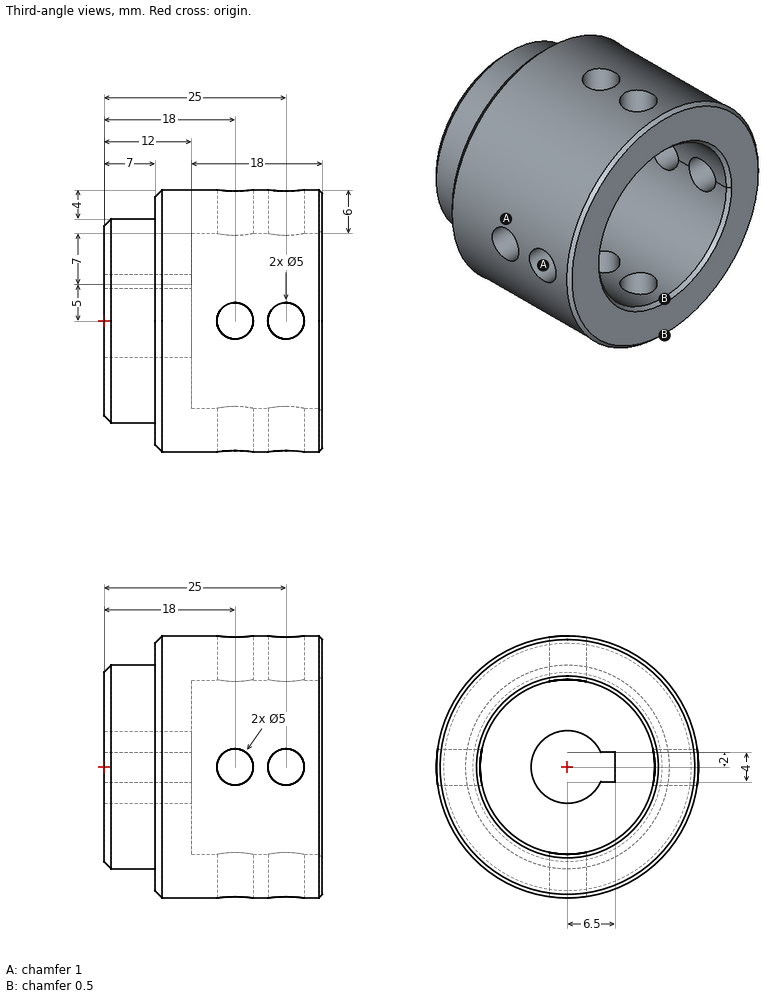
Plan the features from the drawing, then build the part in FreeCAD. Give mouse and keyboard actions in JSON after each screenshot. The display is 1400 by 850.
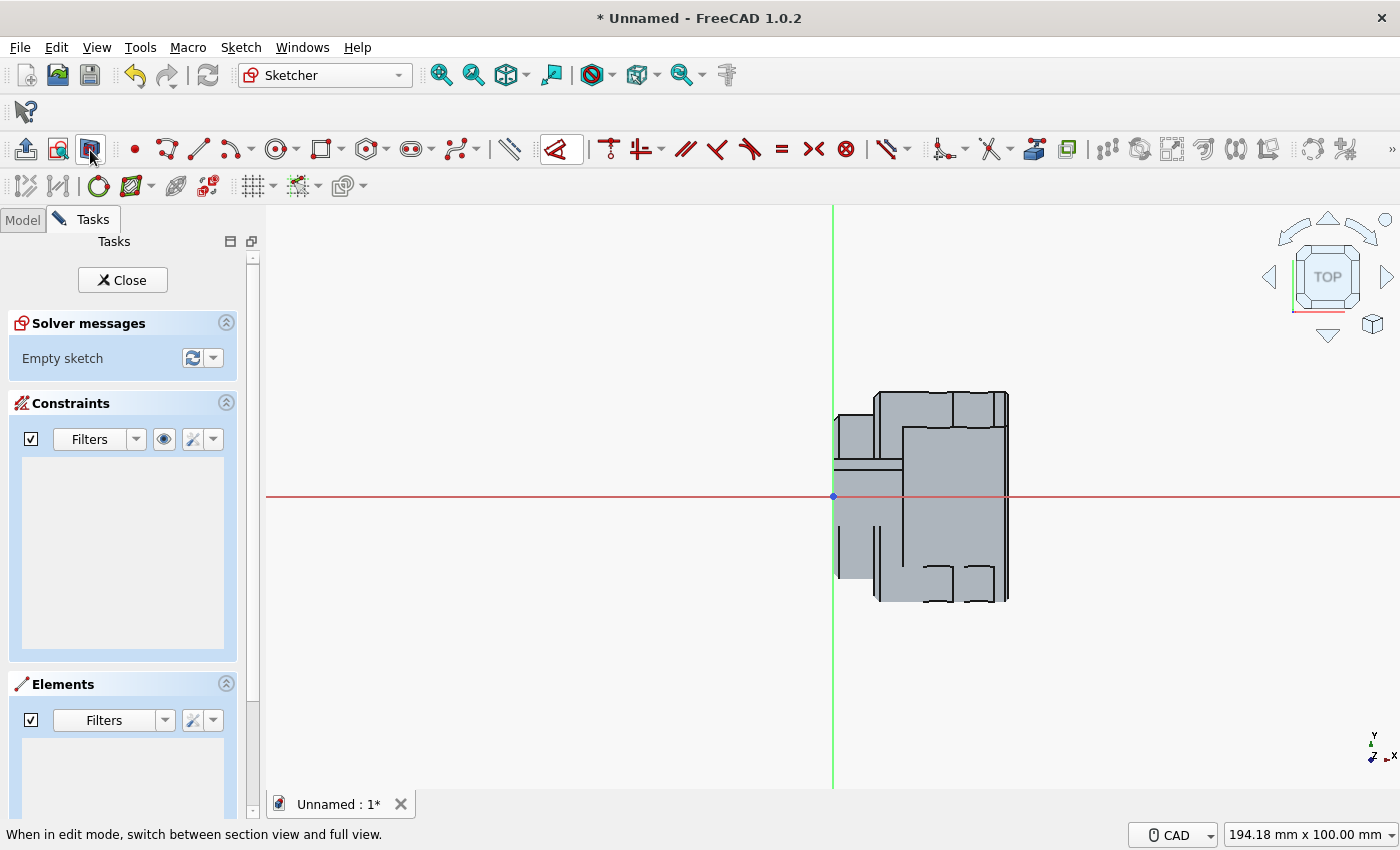
{"action": "scroll", "coordinate": [962, 497], "scroll_direction": "up", "scroll_amount": 7}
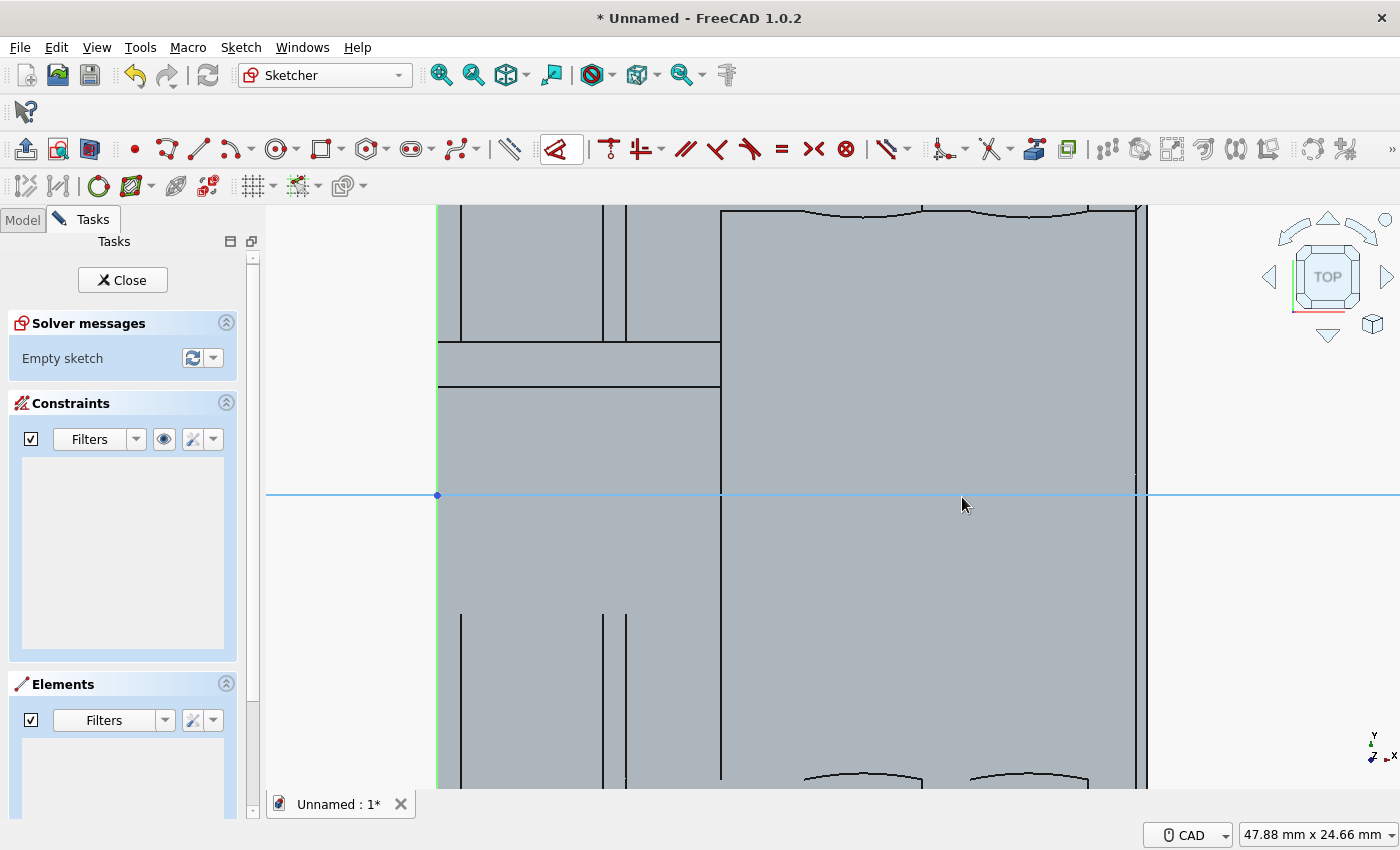
{"action": "left_click", "coordinate": [276, 150]}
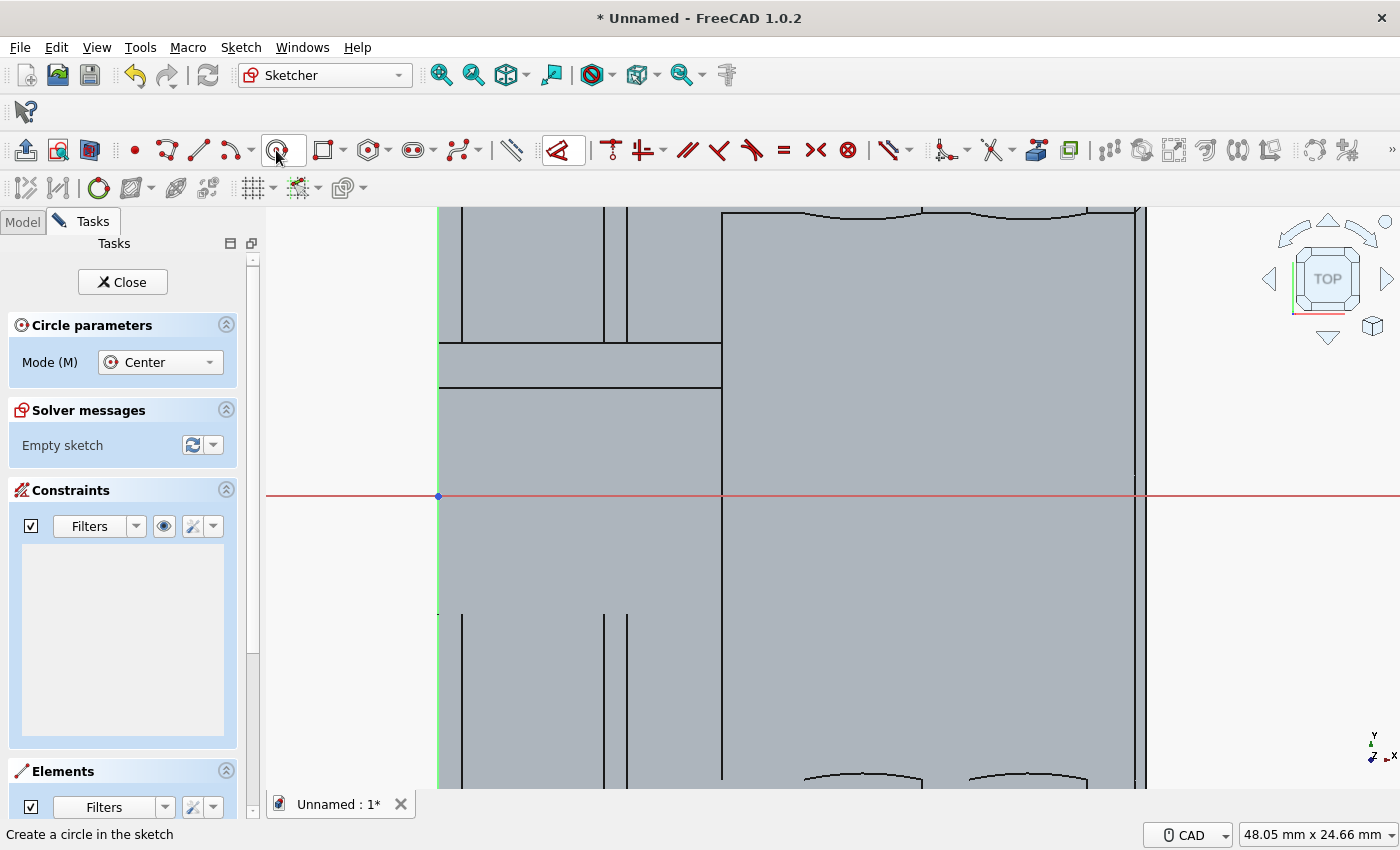
{"action": "left_click", "coordinate": [1028, 496]}
{"action": "left_click", "coordinate": [1070, 455]}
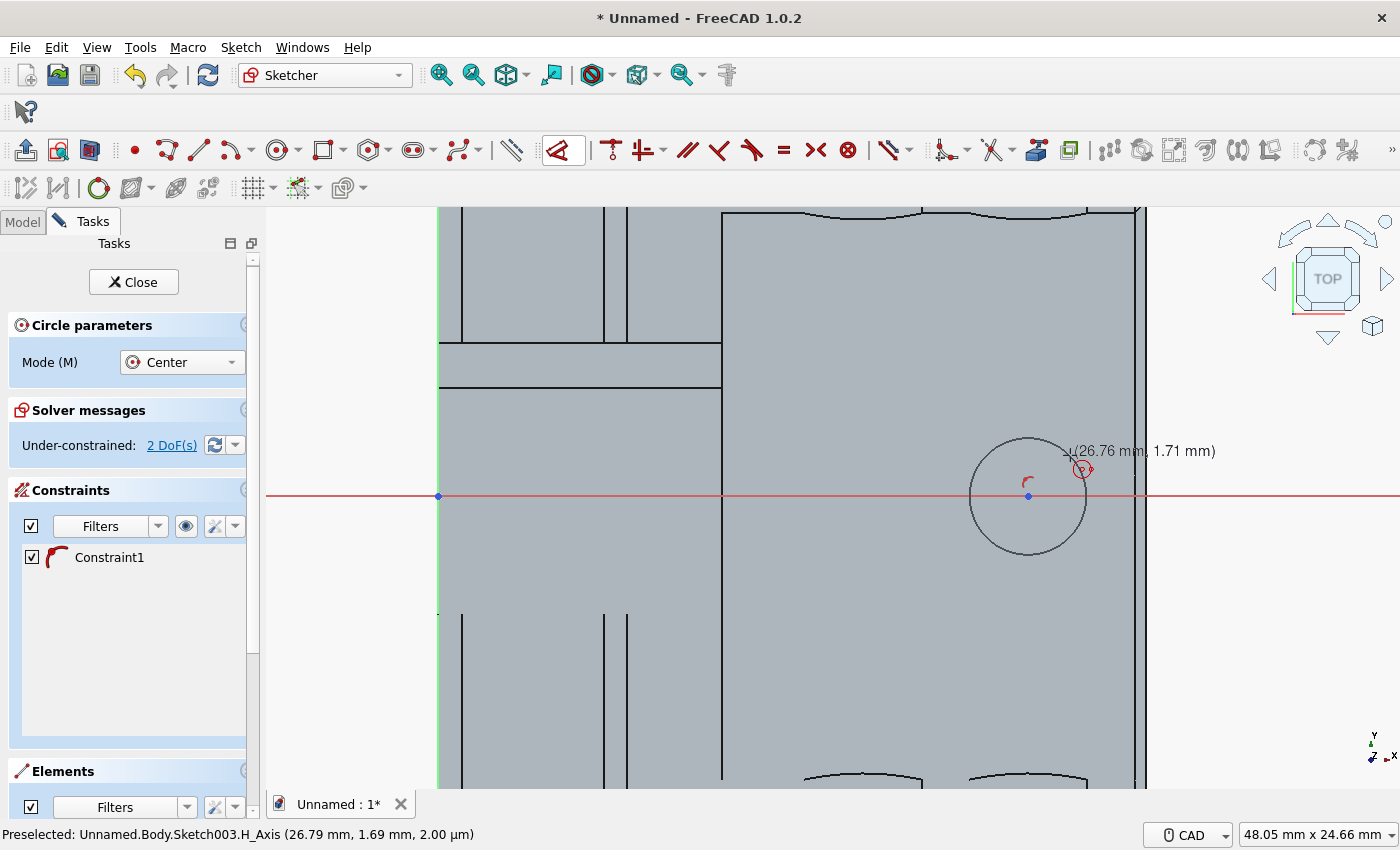
{"action": "left_click", "coordinate": [863, 496]}
{"action": "left_click", "coordinate": [905, 455]}
{"action": "key", "text": "Escape"}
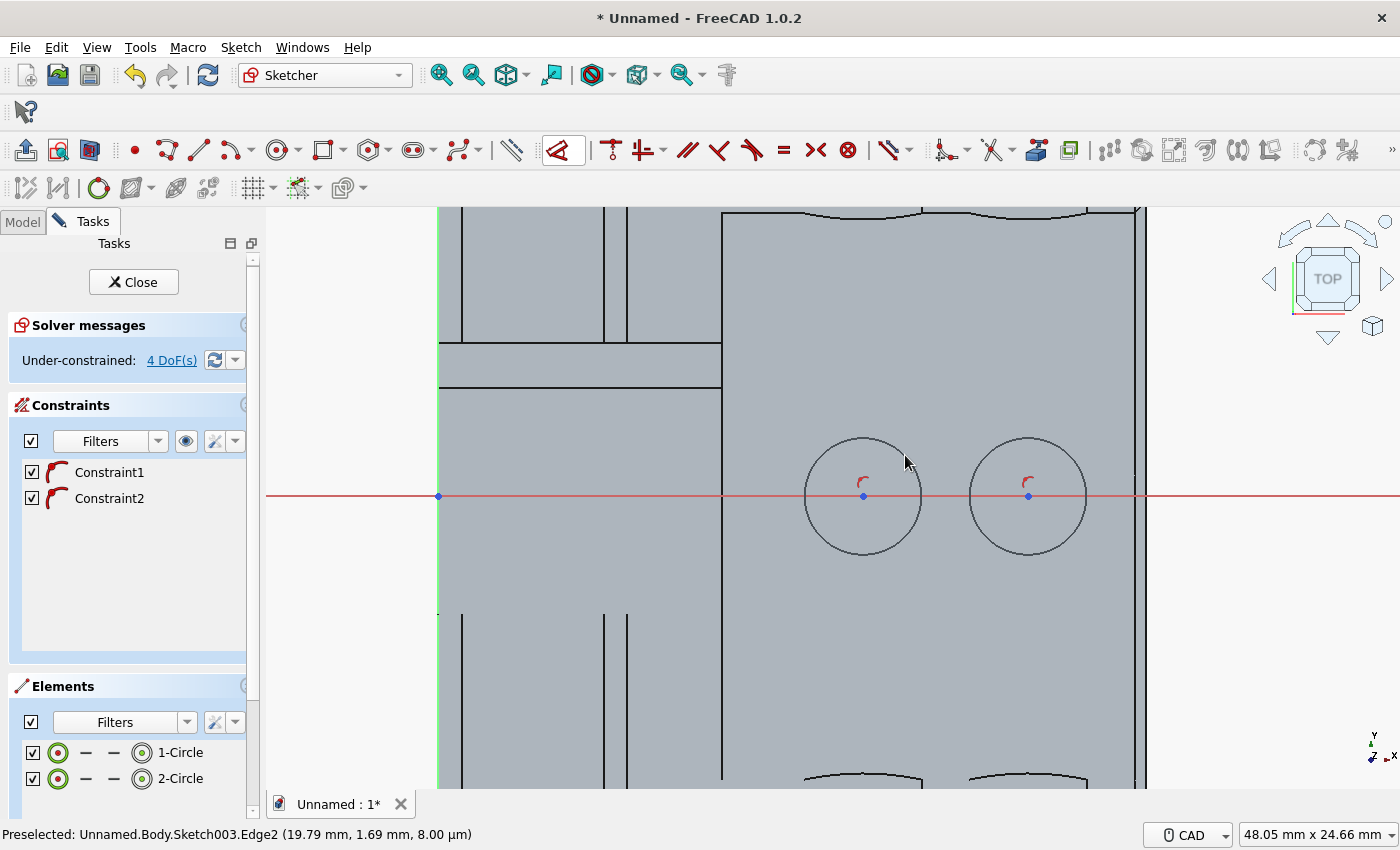
{"action": "left_click", "coordinate": [1069, 455]}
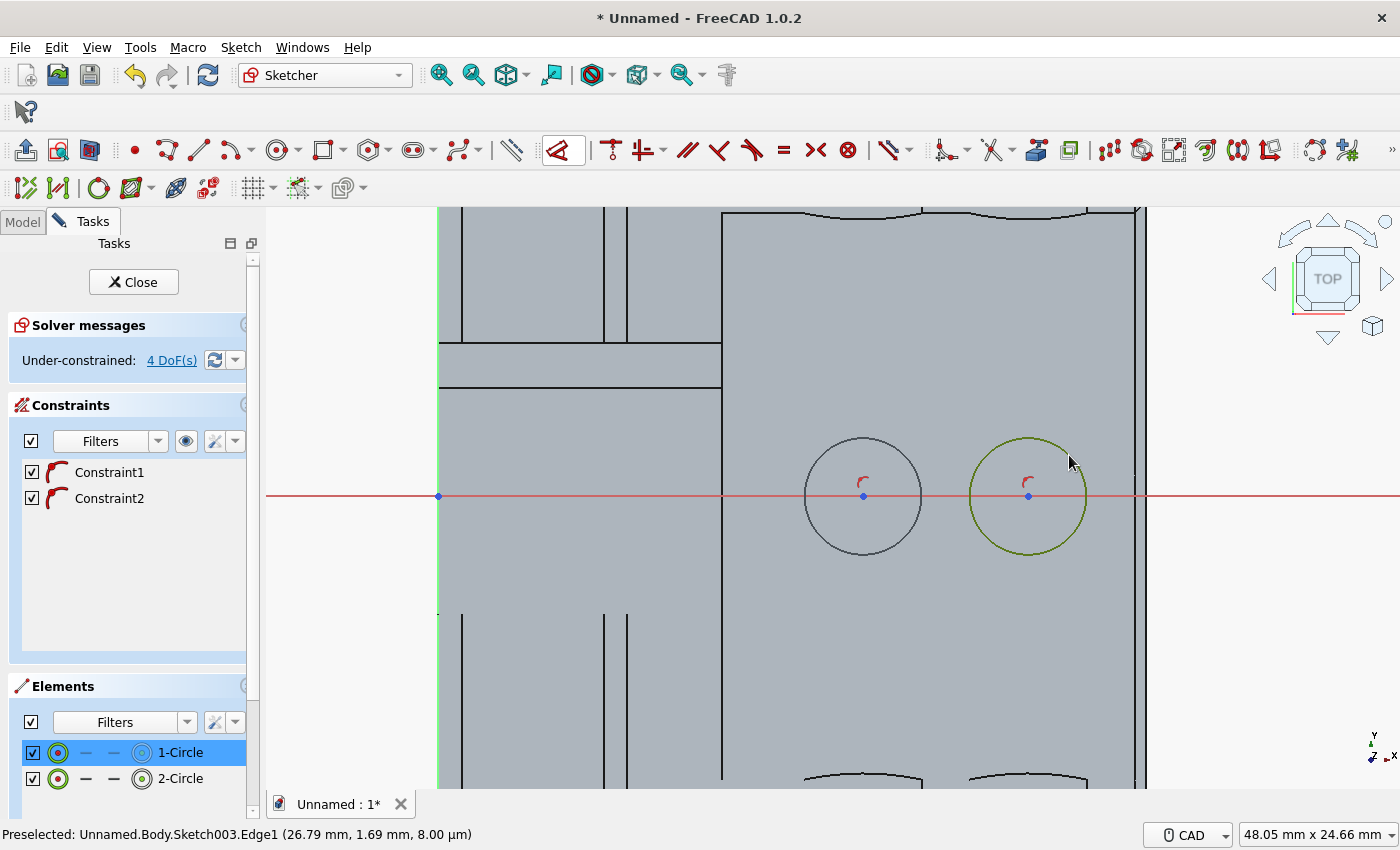
{"action": "left_click", "coordinate": [904, 455]}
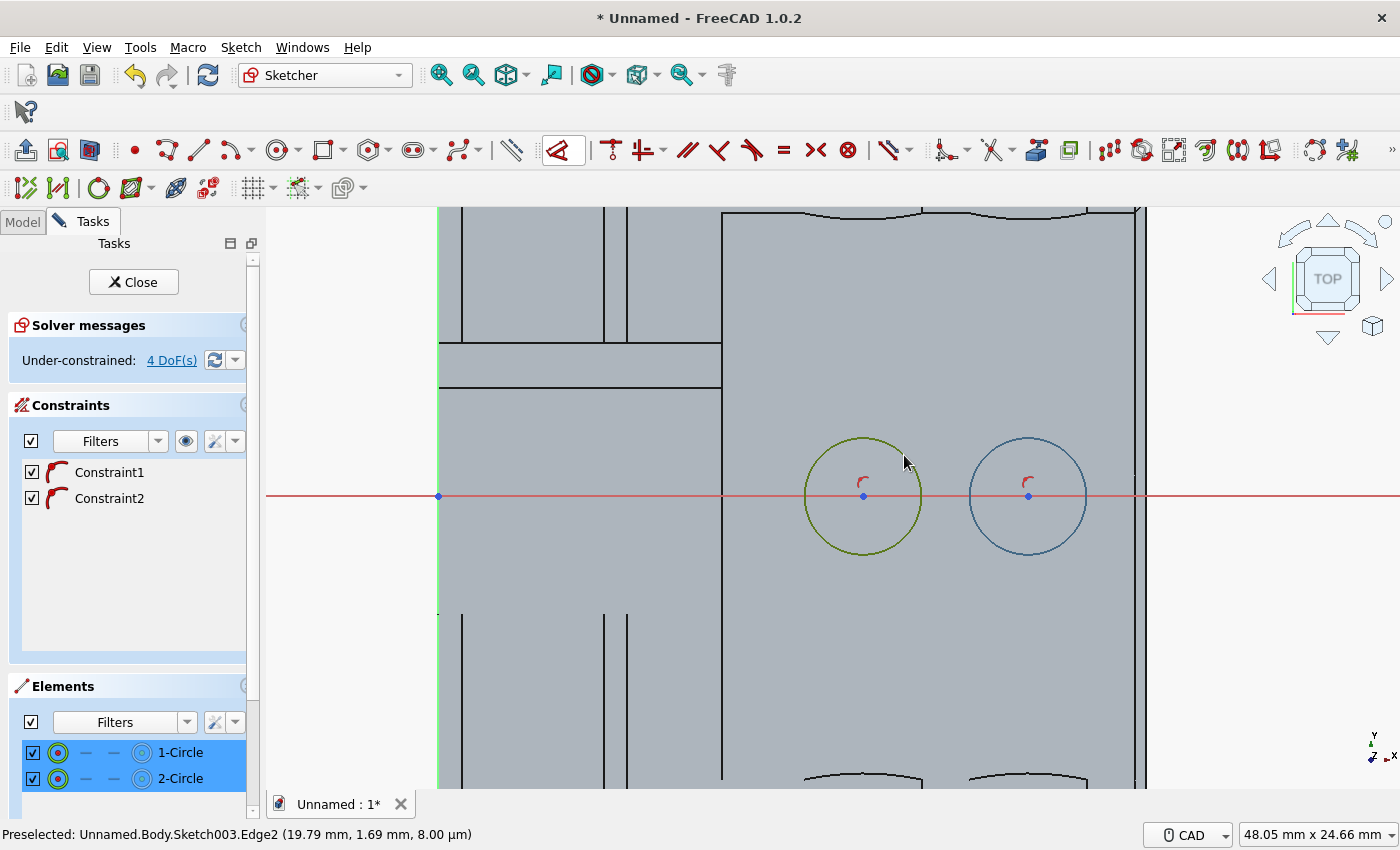
{"action": "left_click", "coordinate": [784, 150]}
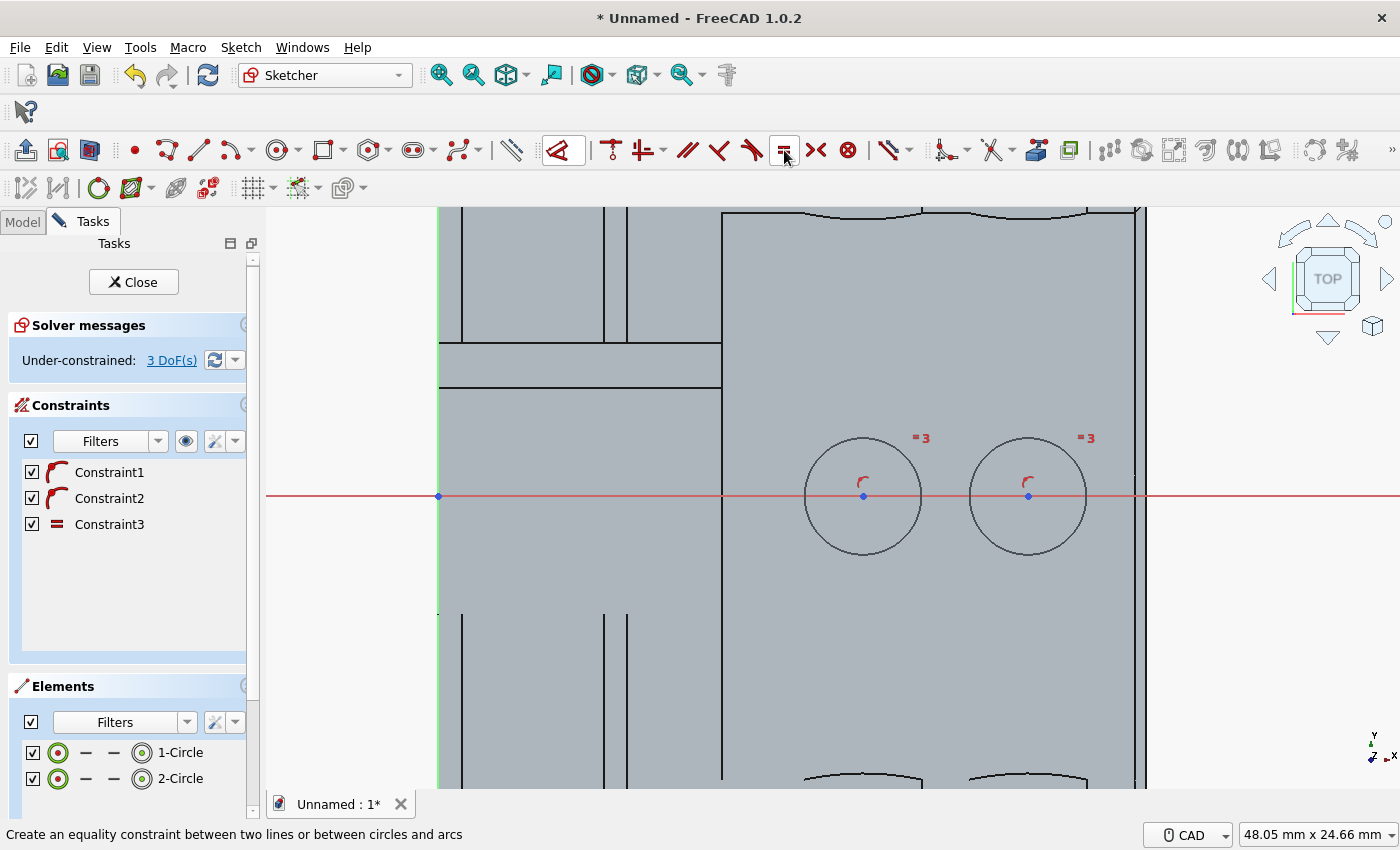
{"action": "left_click", "coordinate": [1069, 455]}